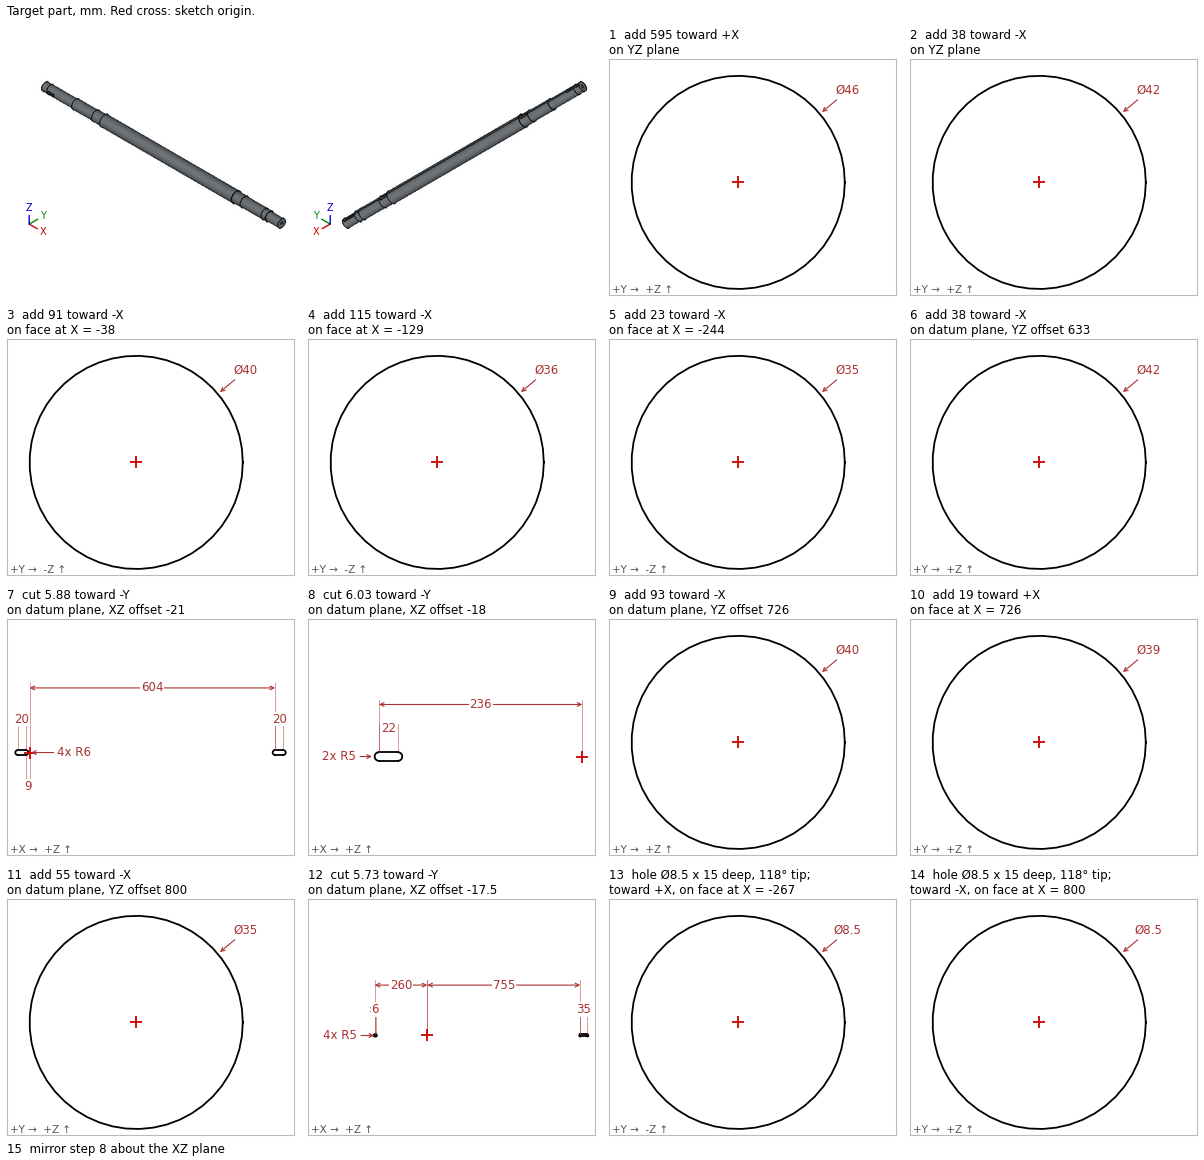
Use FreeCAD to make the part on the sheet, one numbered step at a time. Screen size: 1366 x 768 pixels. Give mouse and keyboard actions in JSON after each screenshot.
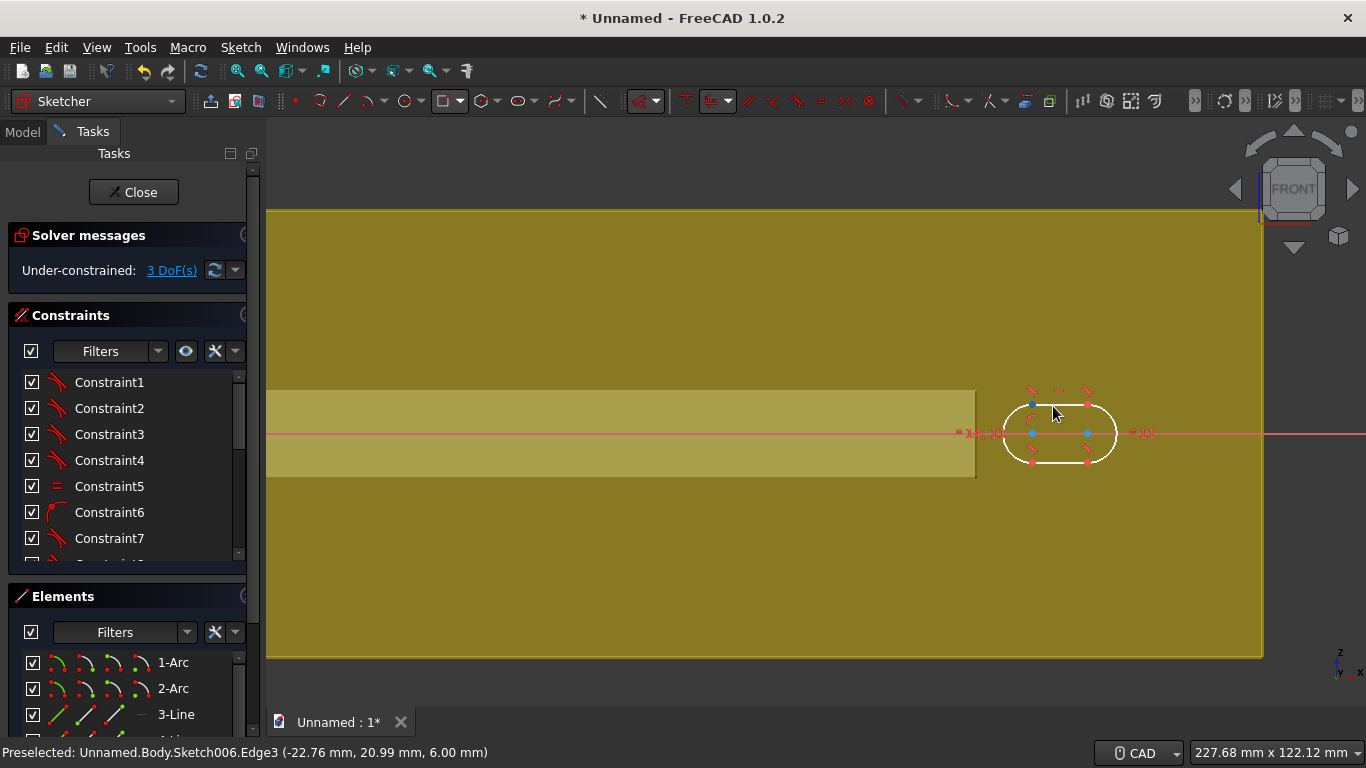
{"action": "left_click", "coordinate": [1049, 405]}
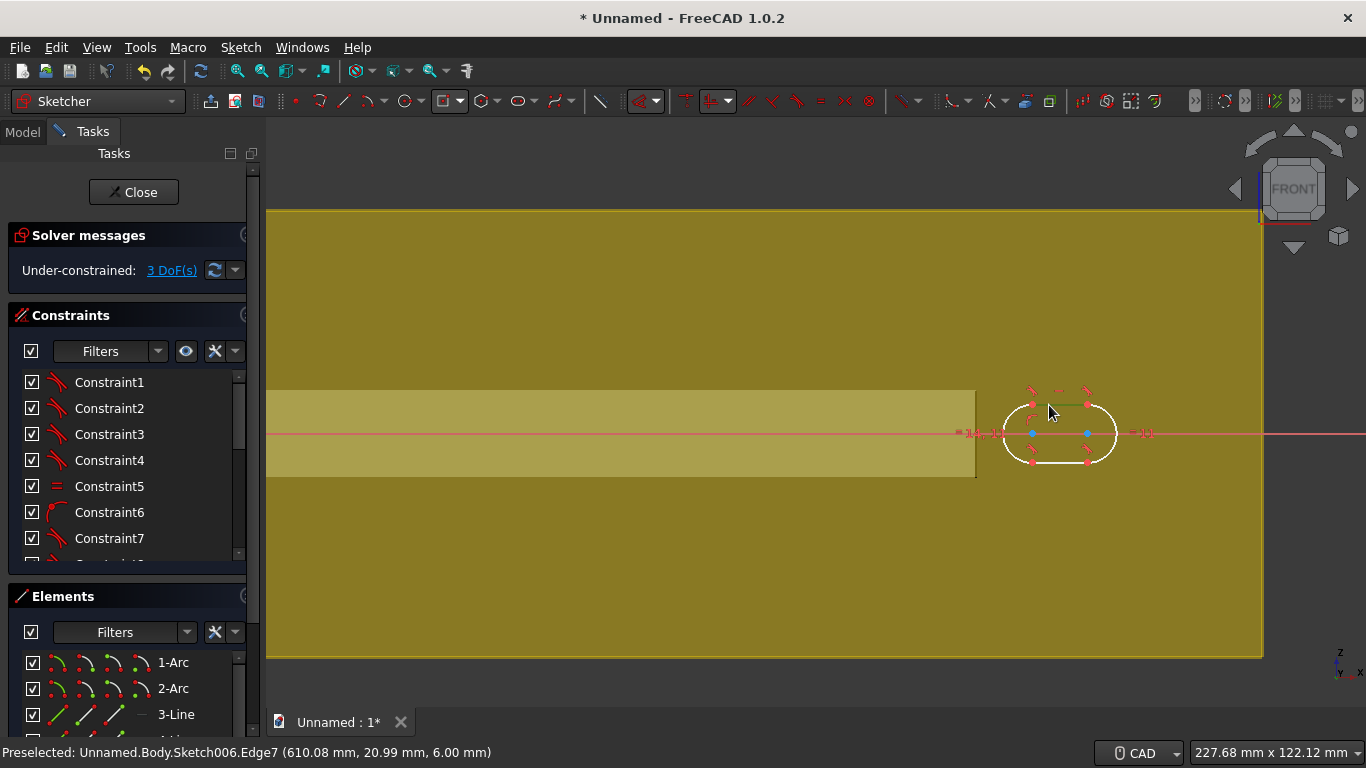
{"action": "key", "text": "l"}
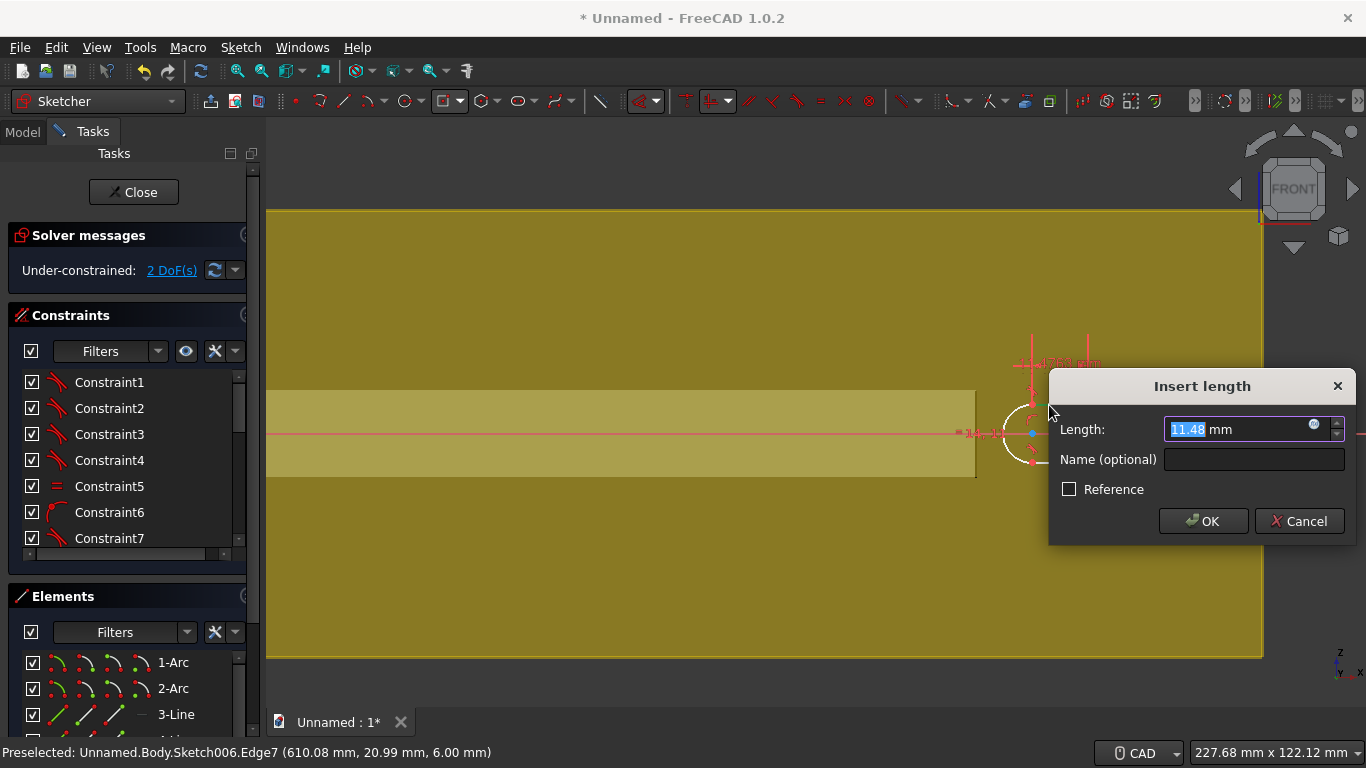
{"action": "type", "text": "20"}
{"action": "key", "text": "Return"}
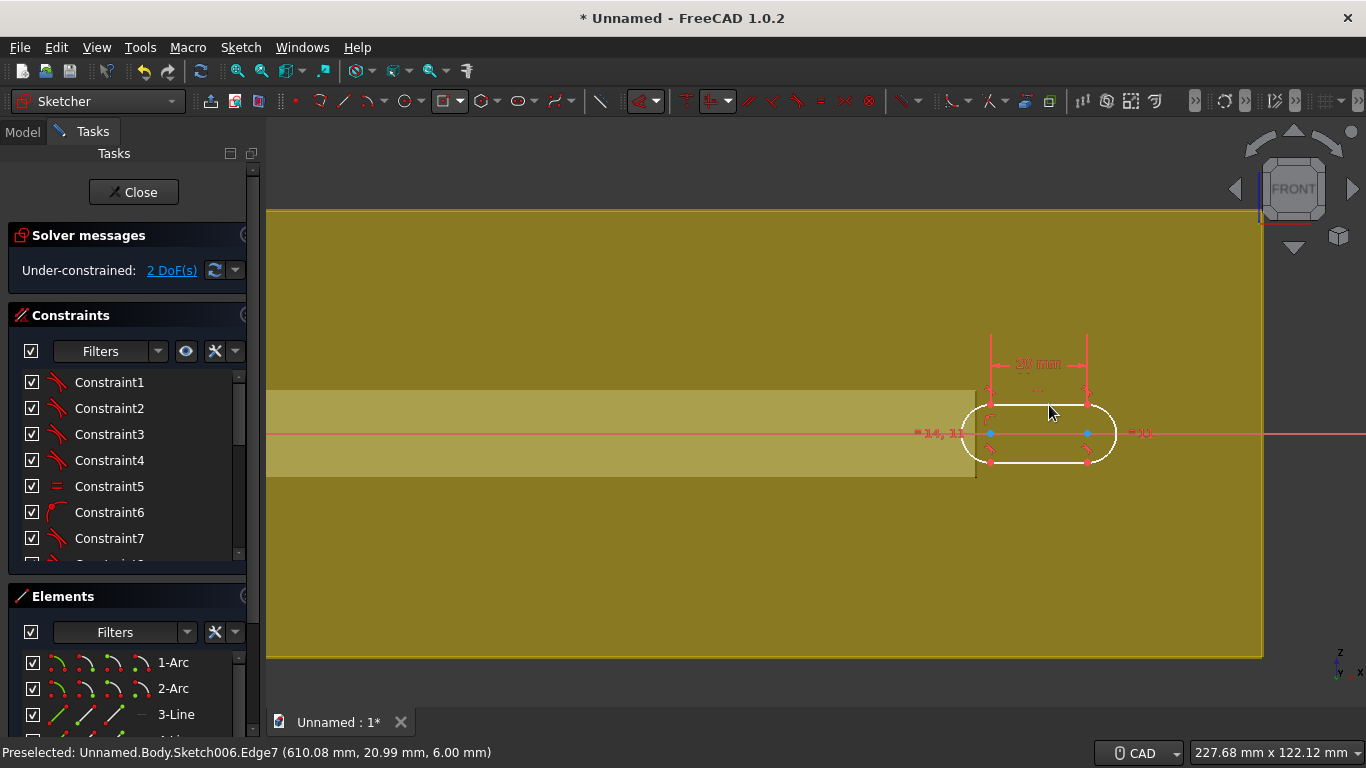
{"action": "scroll", "coordinate": [1053, 406], "scroll_direction": "down", "scroll_amount": 8}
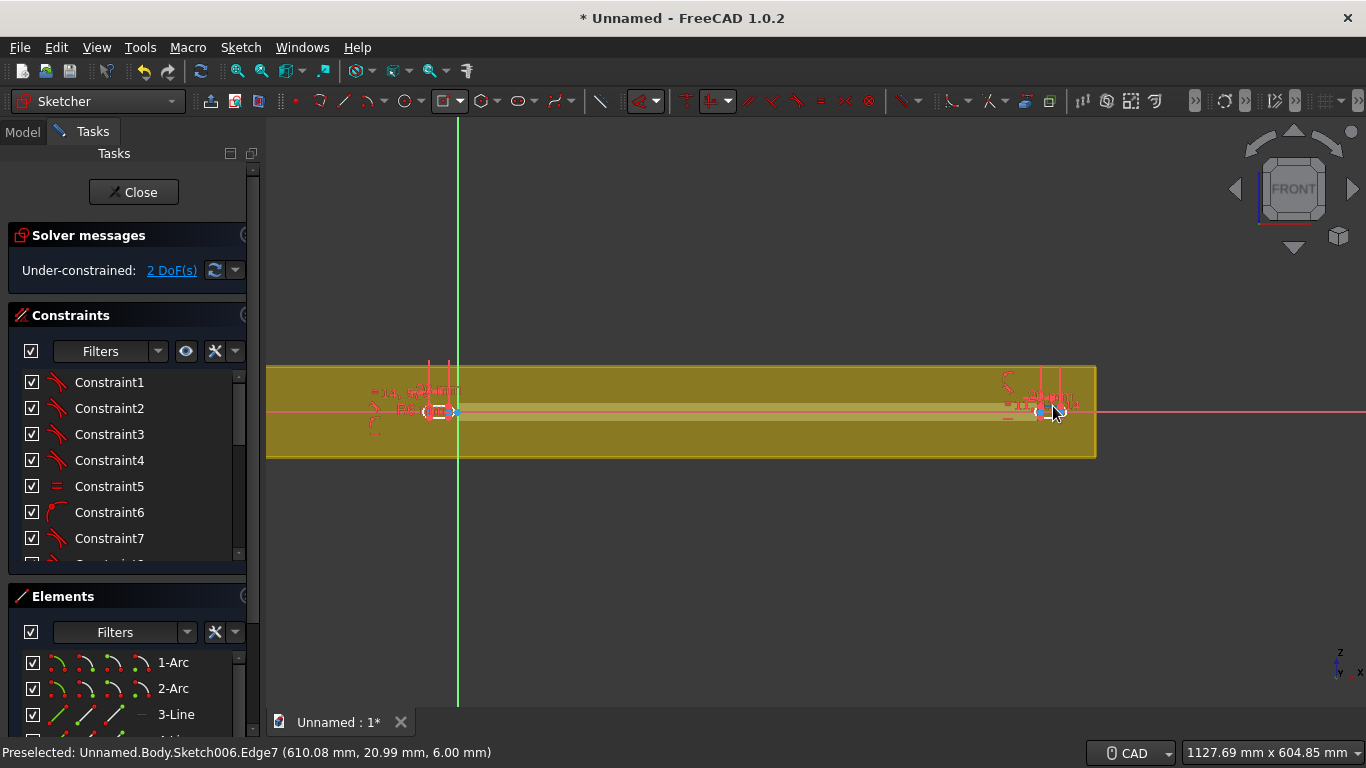
{"action": "scroll", "coordinate": [449, 418], "scroll_direction": "up", "scroll_amount": 8}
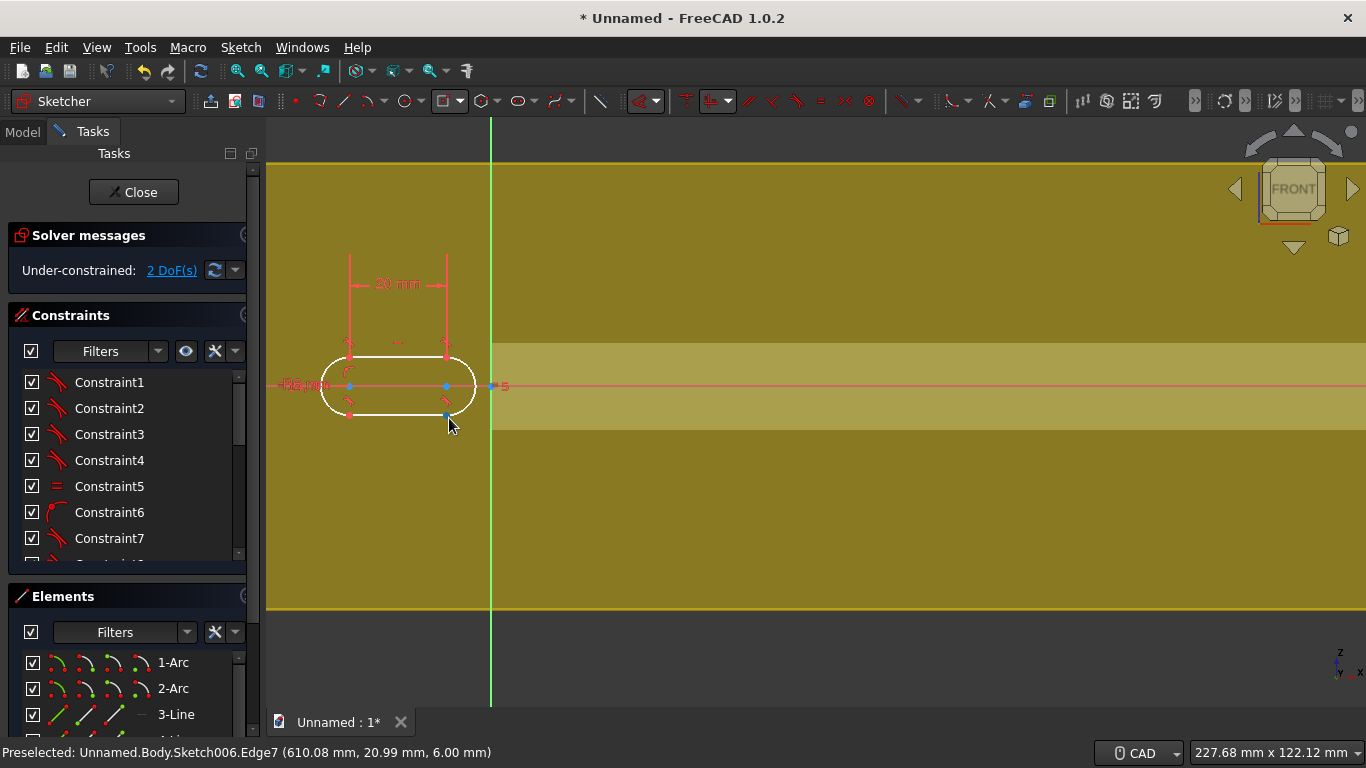
{"action": "left_click", "coordinate": [447, 415]}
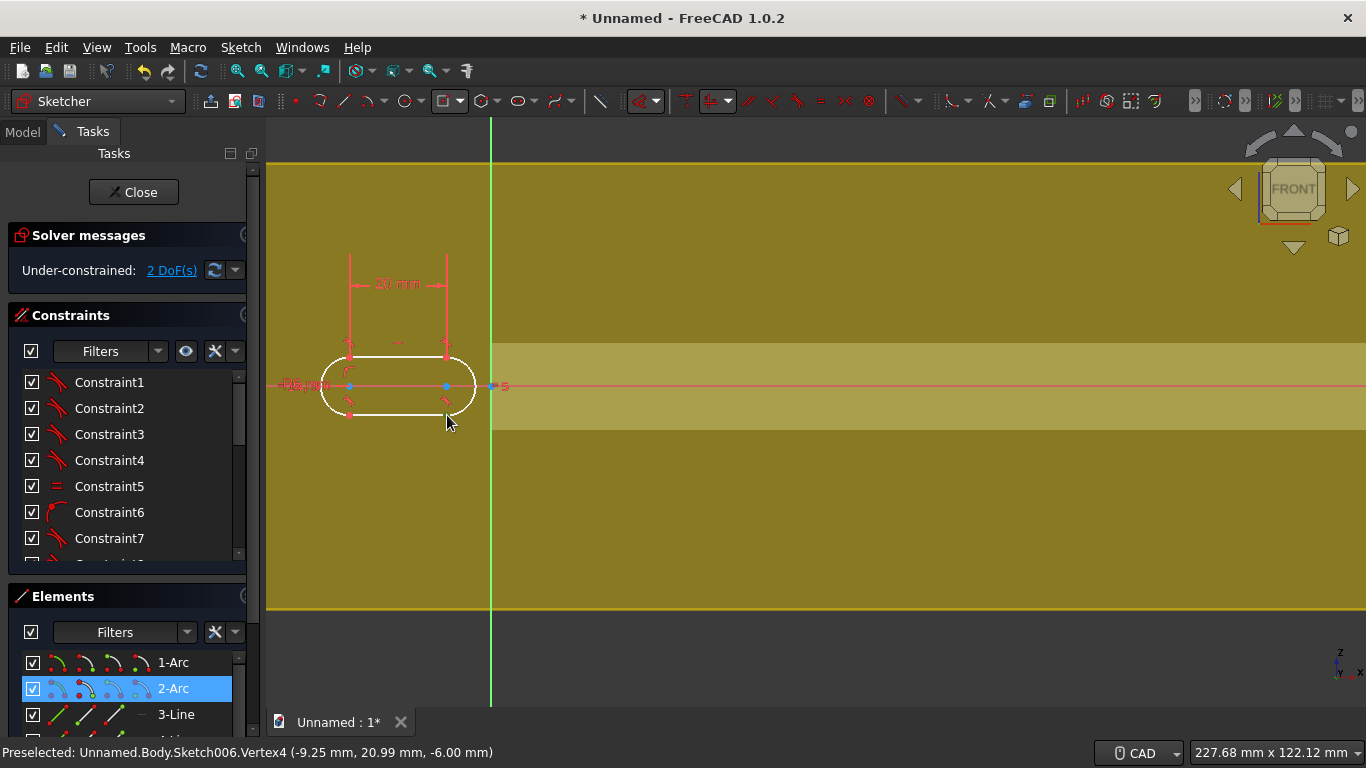
{"action": "left_click", "coordinate": [658, 102]}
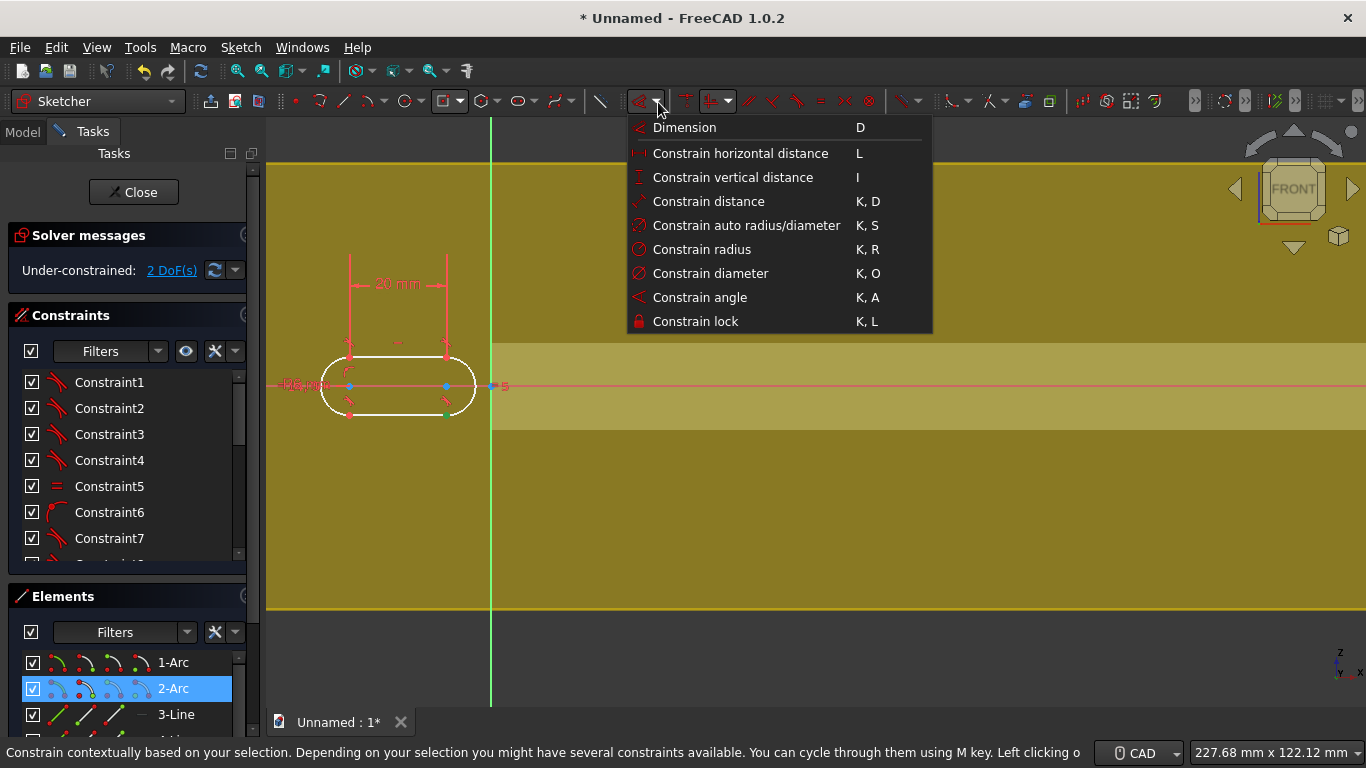
{"action": "left_click", "coordinate": [780, 153]}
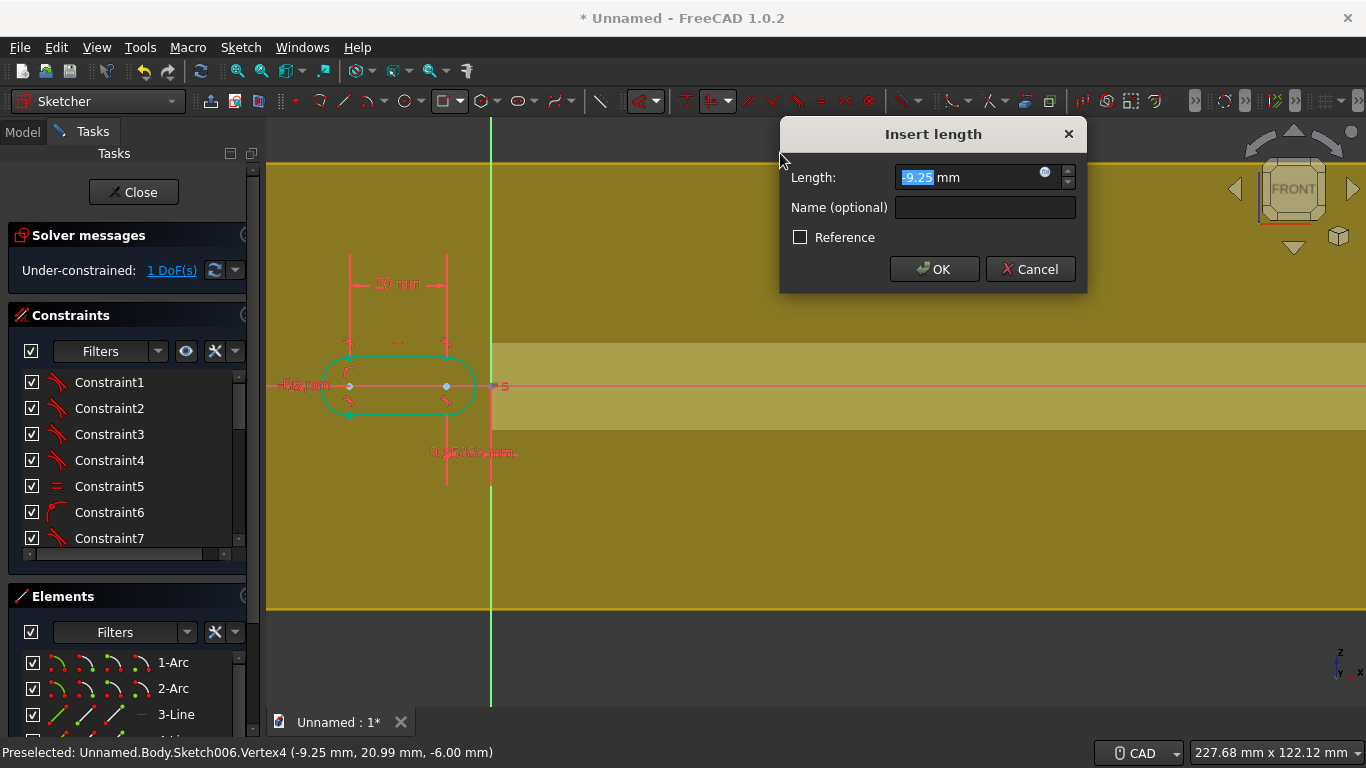
{"action": "type", "text": "-9"}
{"action": "key", "text": "Return"}